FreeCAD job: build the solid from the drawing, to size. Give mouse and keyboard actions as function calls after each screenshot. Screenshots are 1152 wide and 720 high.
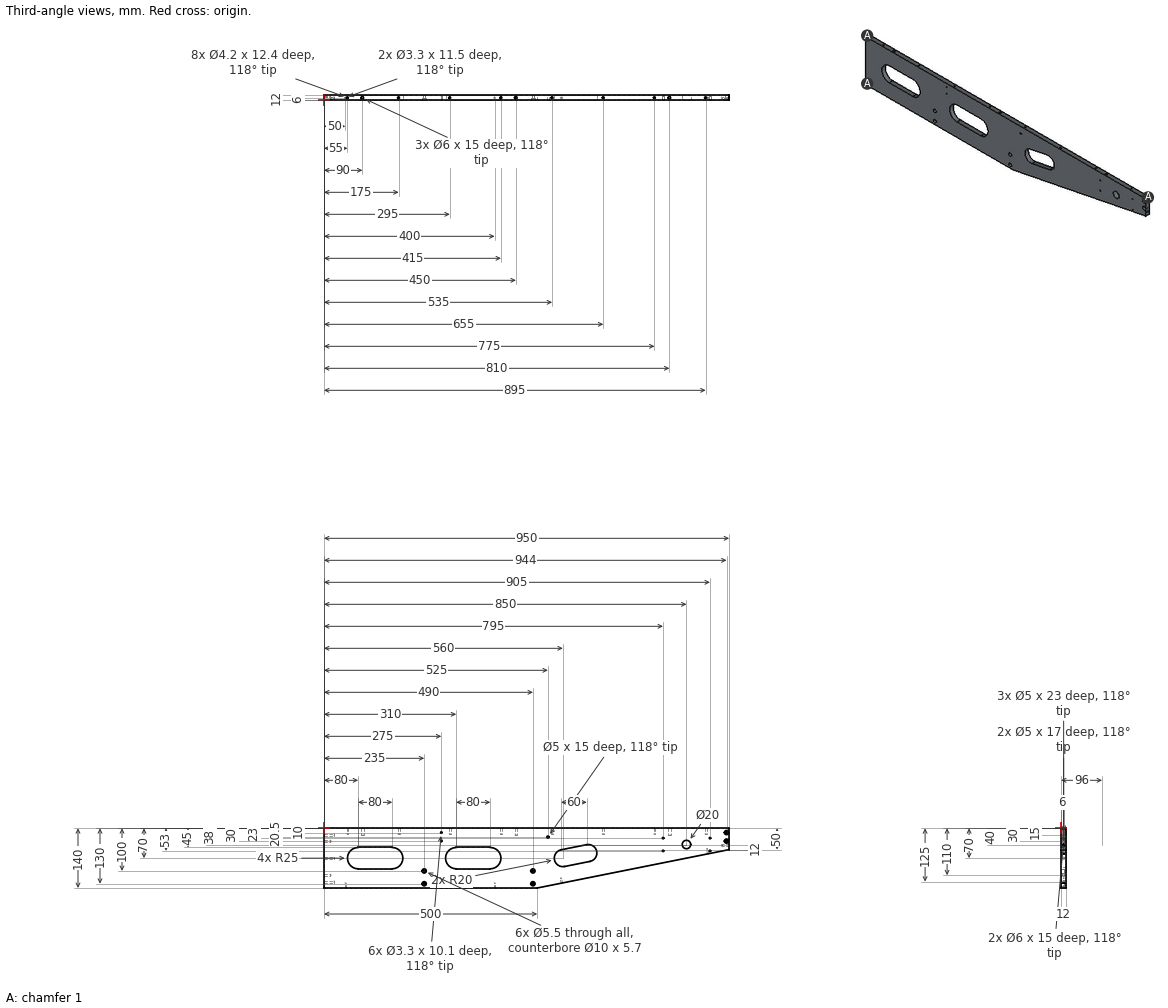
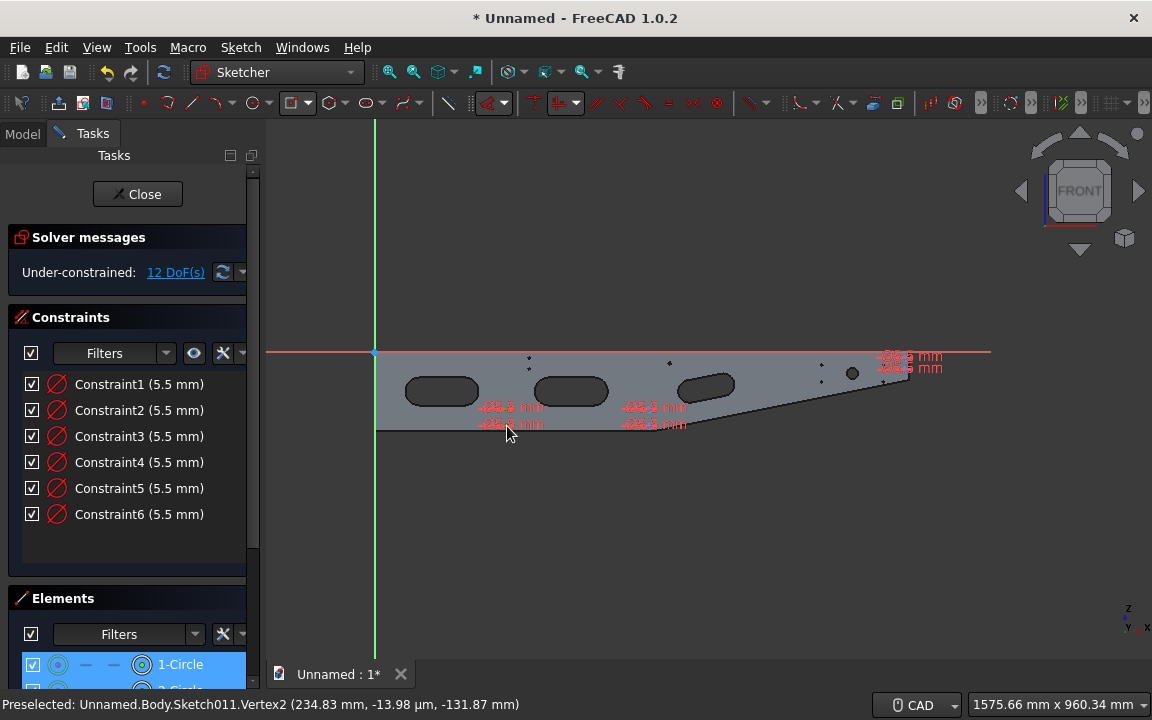
key(v)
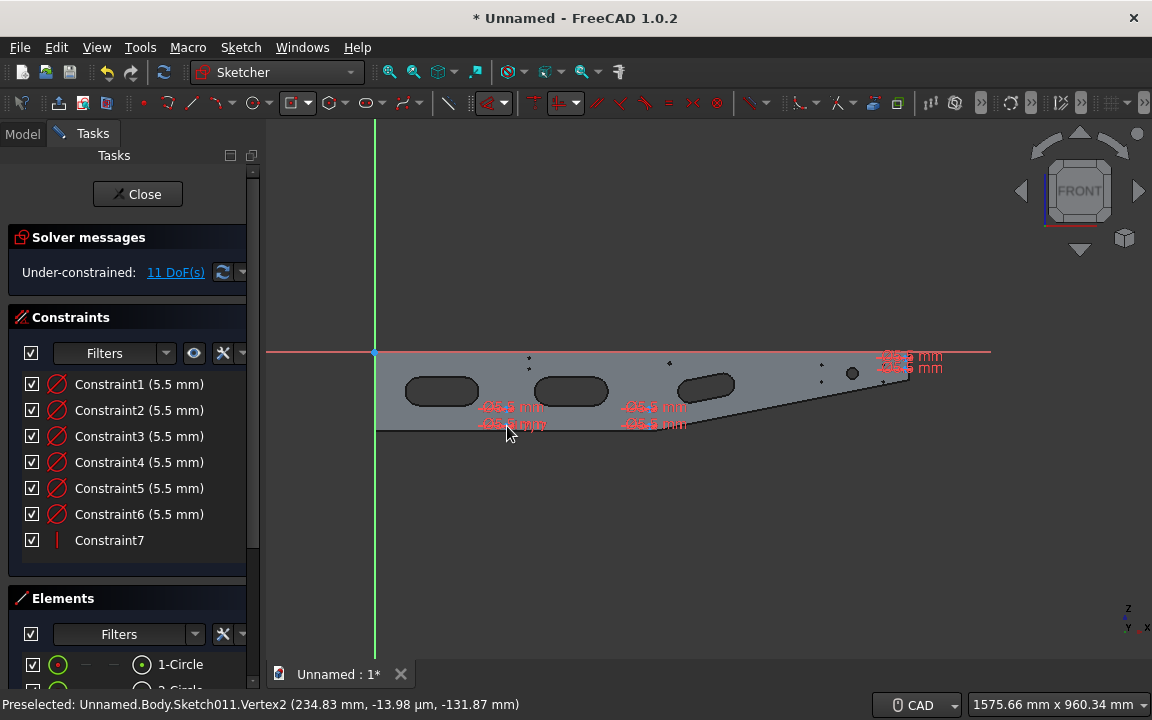
click(507, 409)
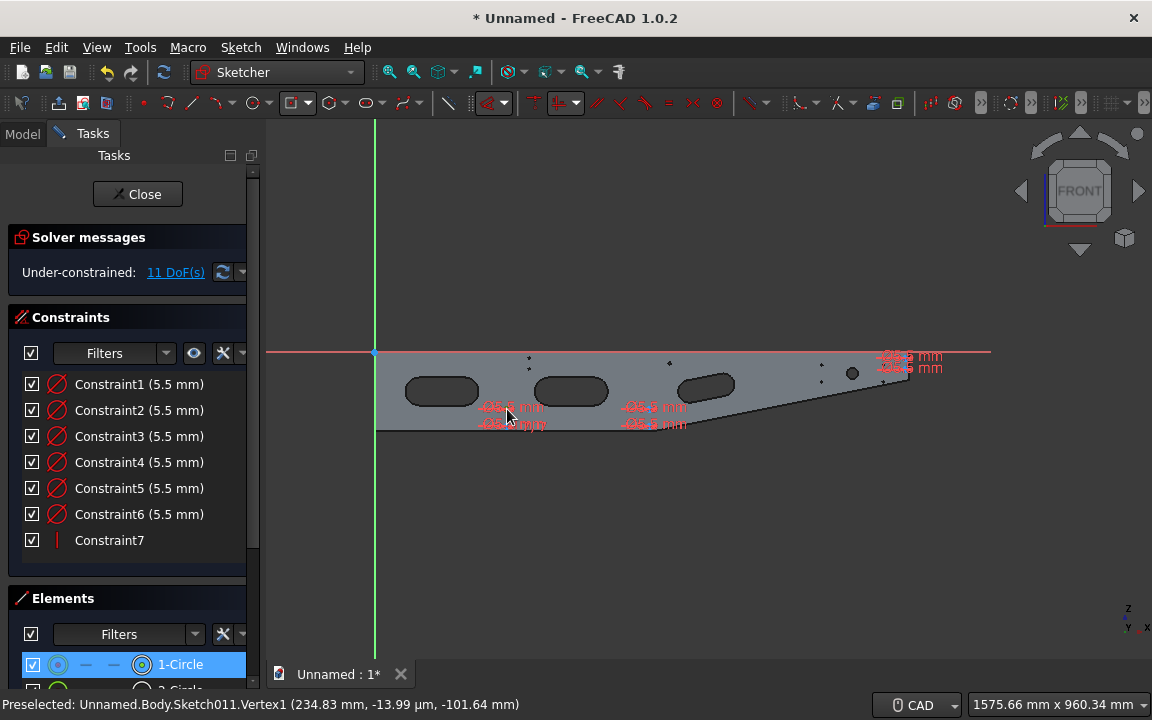
click(650, 409)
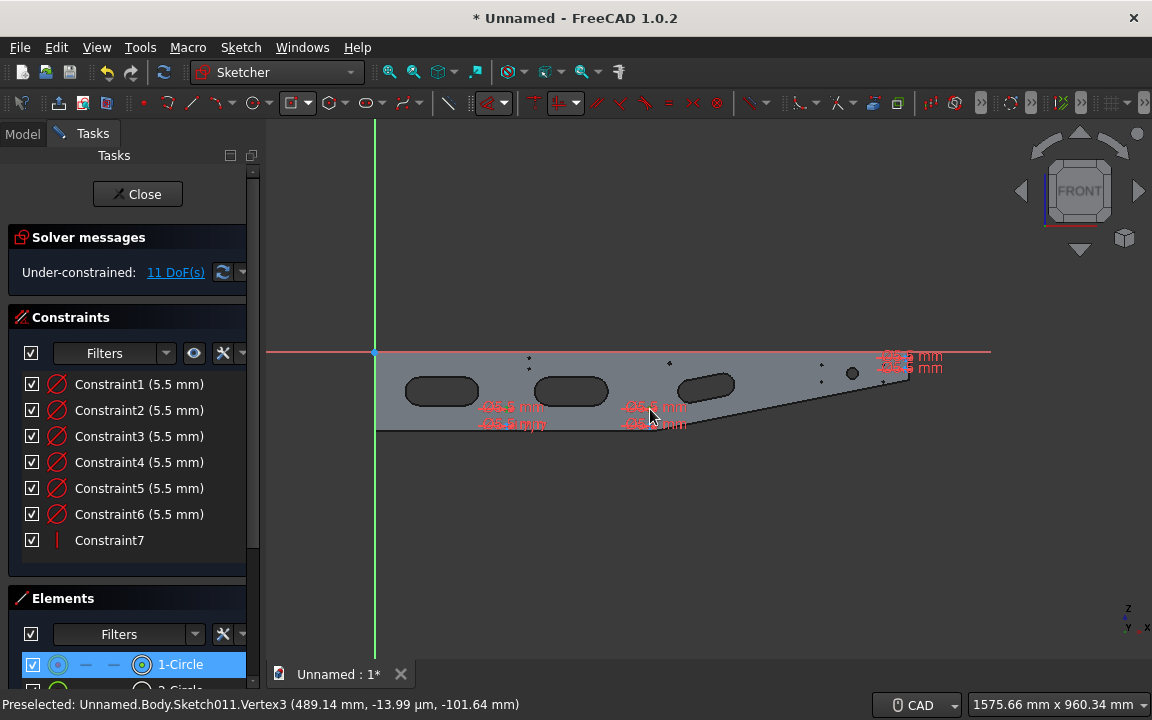
click(578, 104)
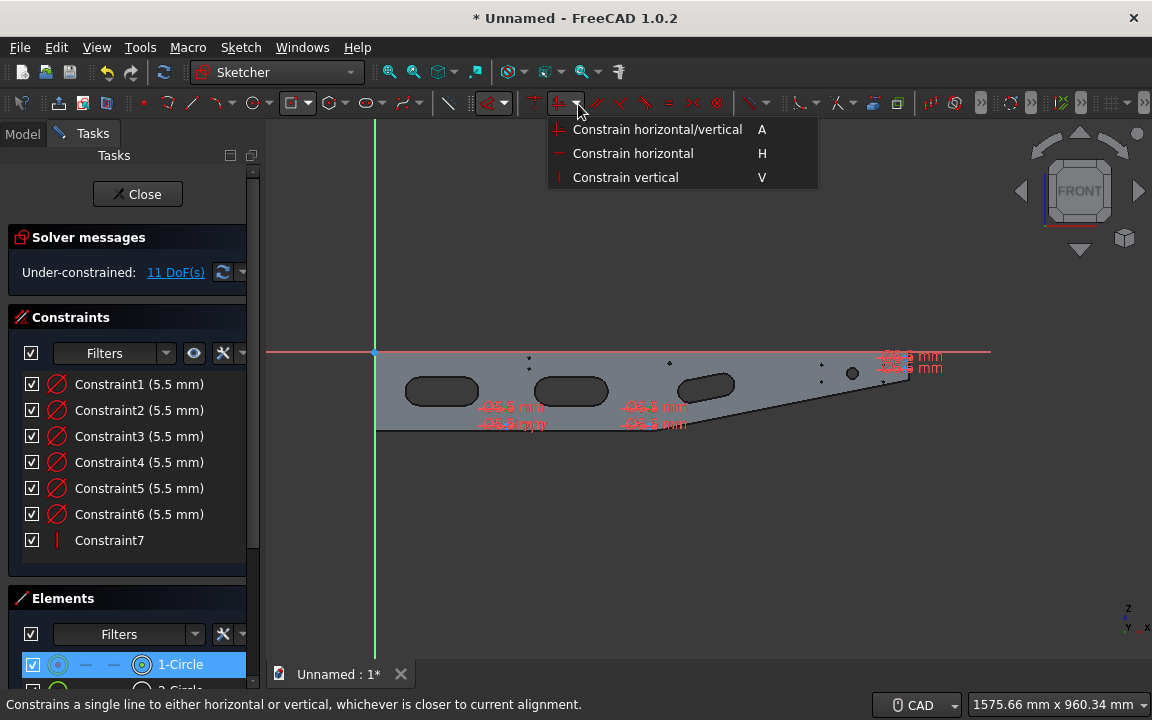
click(683, 153)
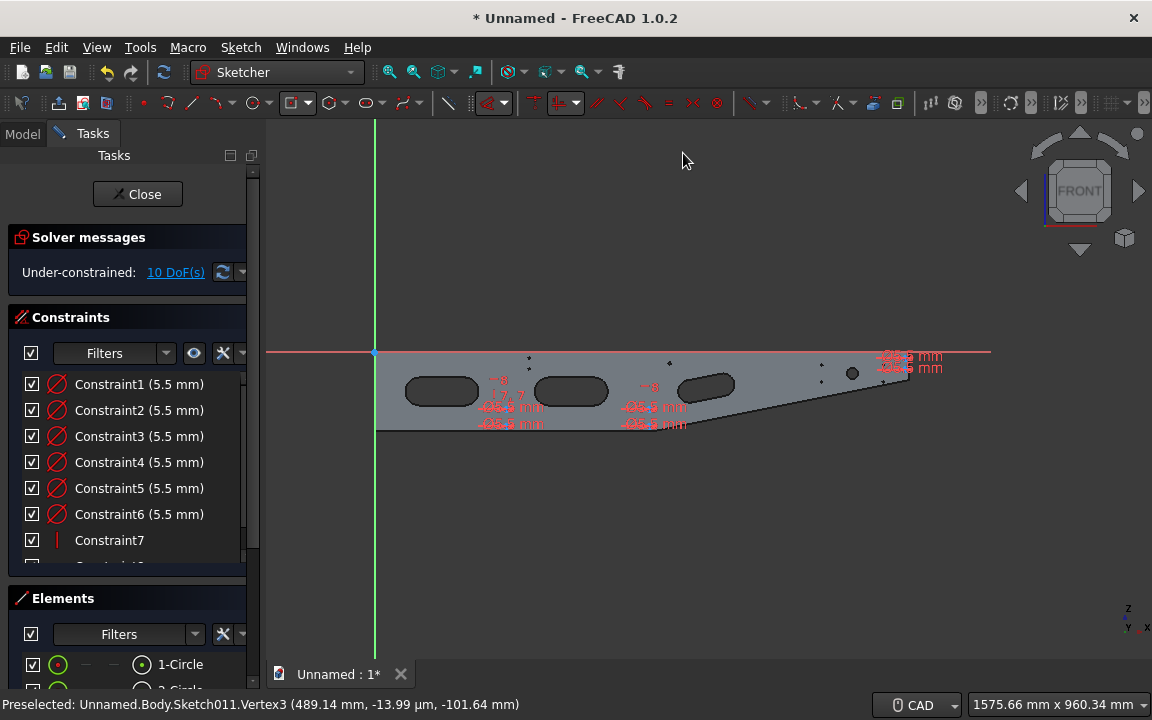
click(650, 409)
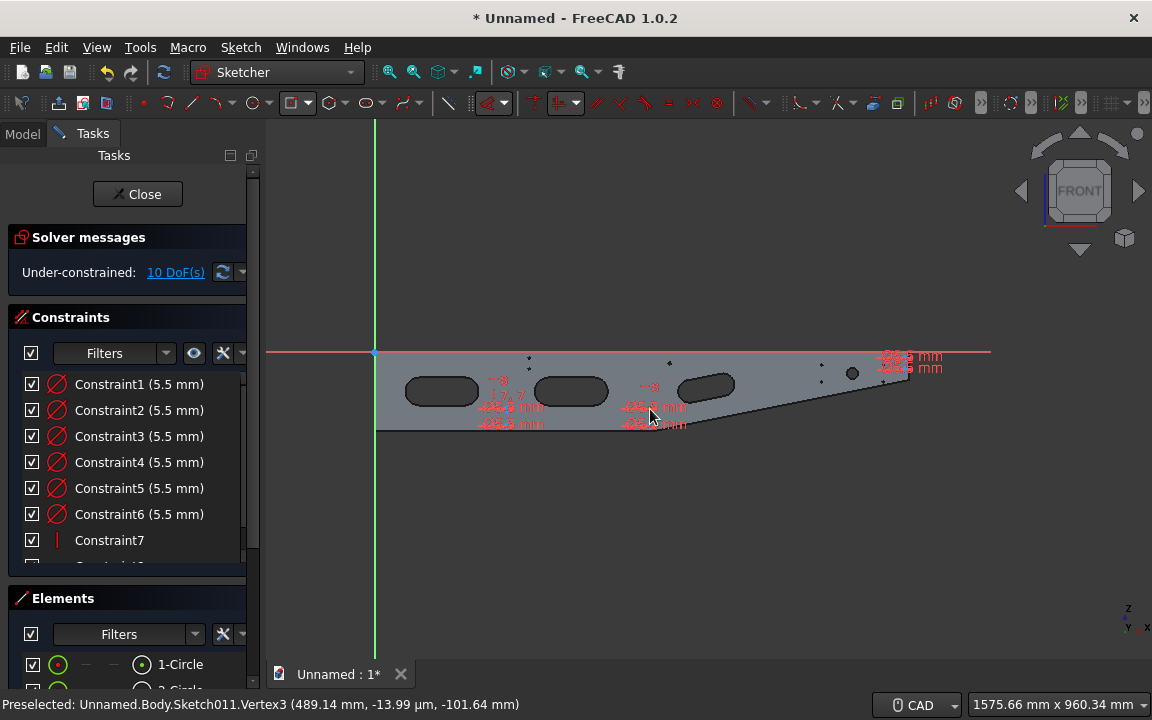
click(650, 426)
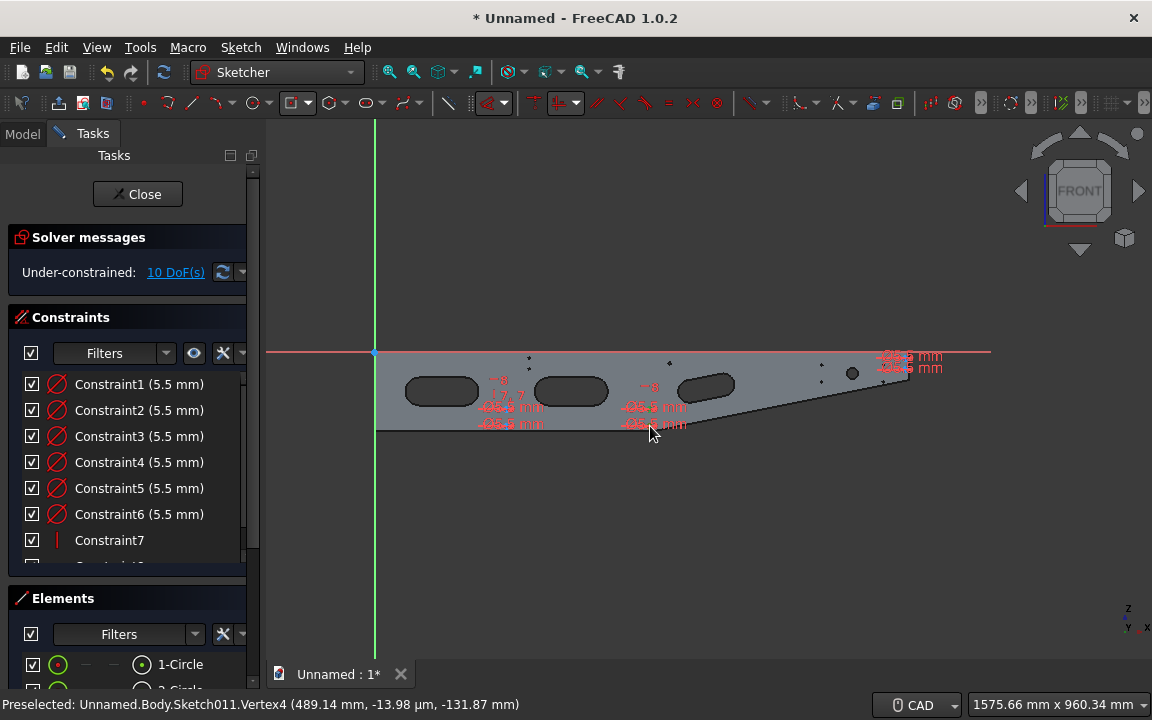
key(v)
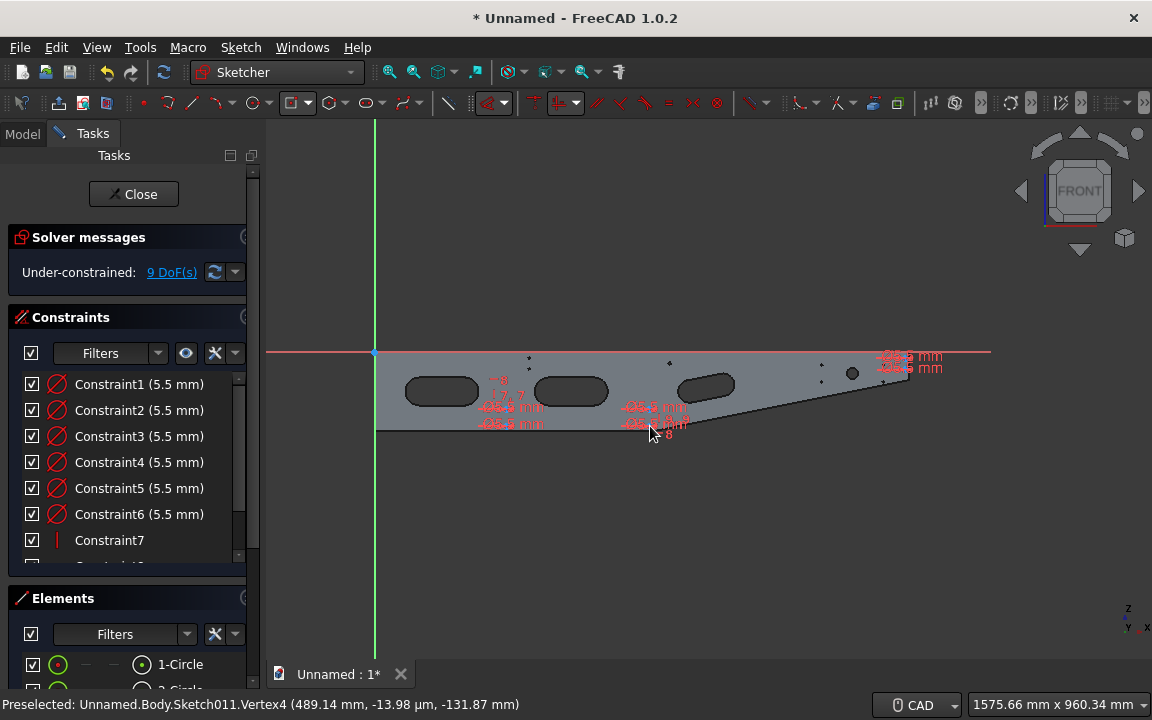
click(507, 426)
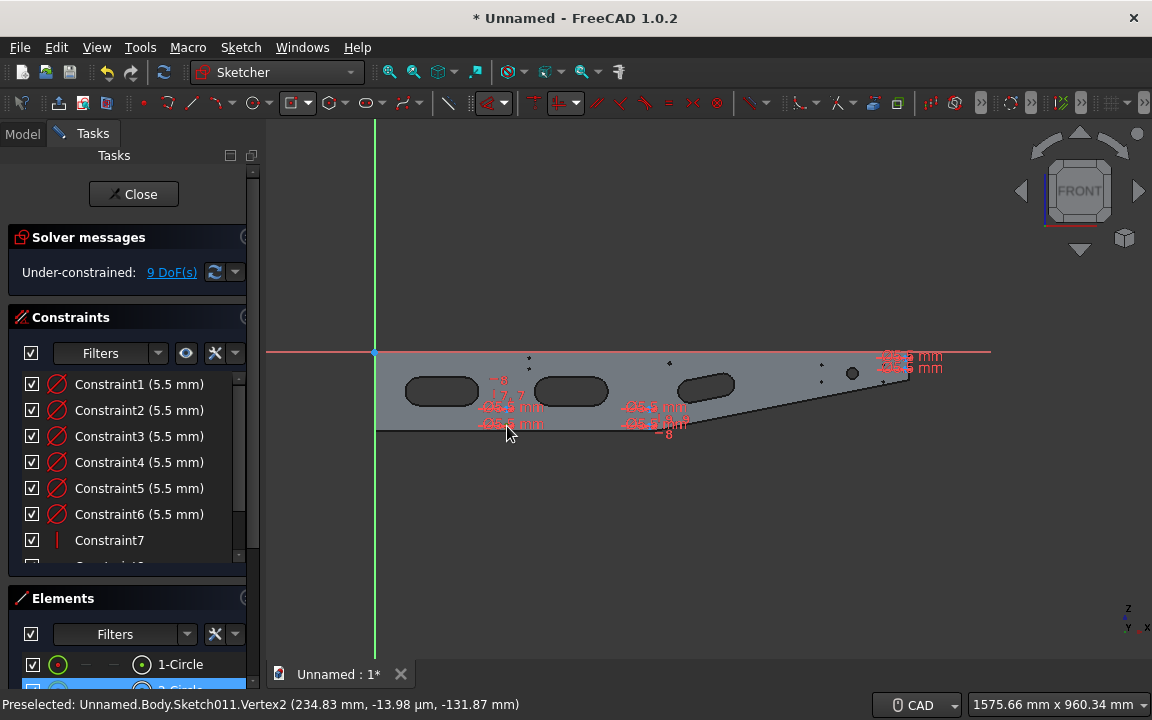
click(650, 426)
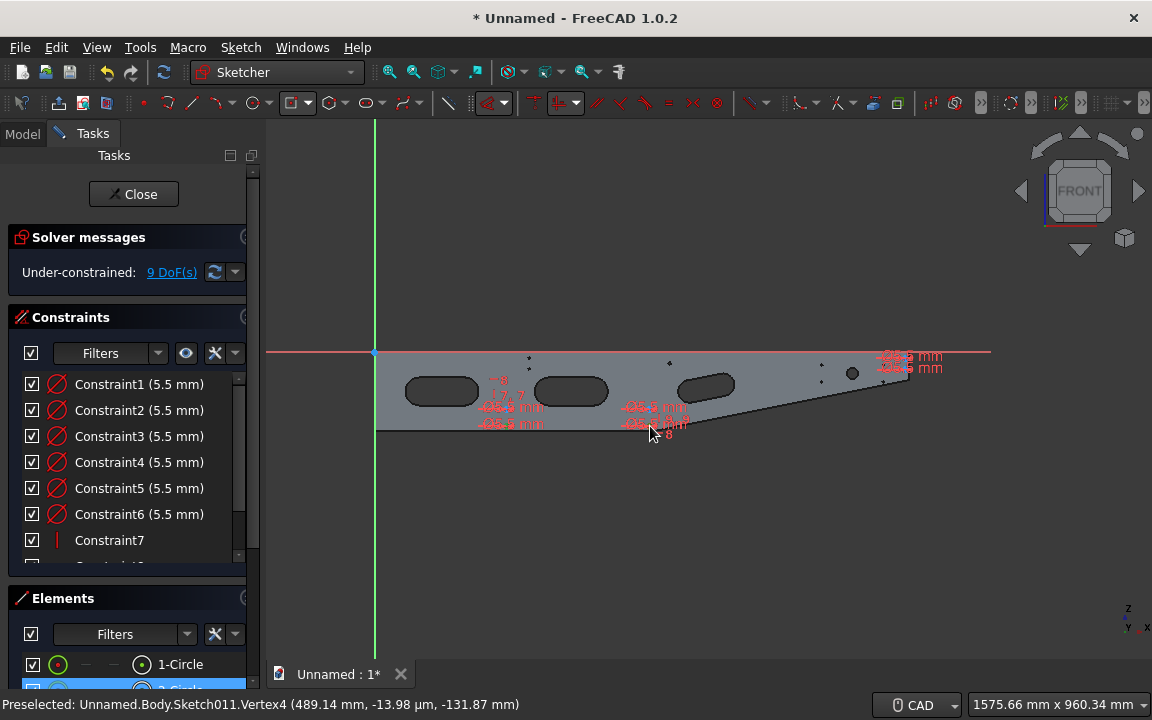
key(h)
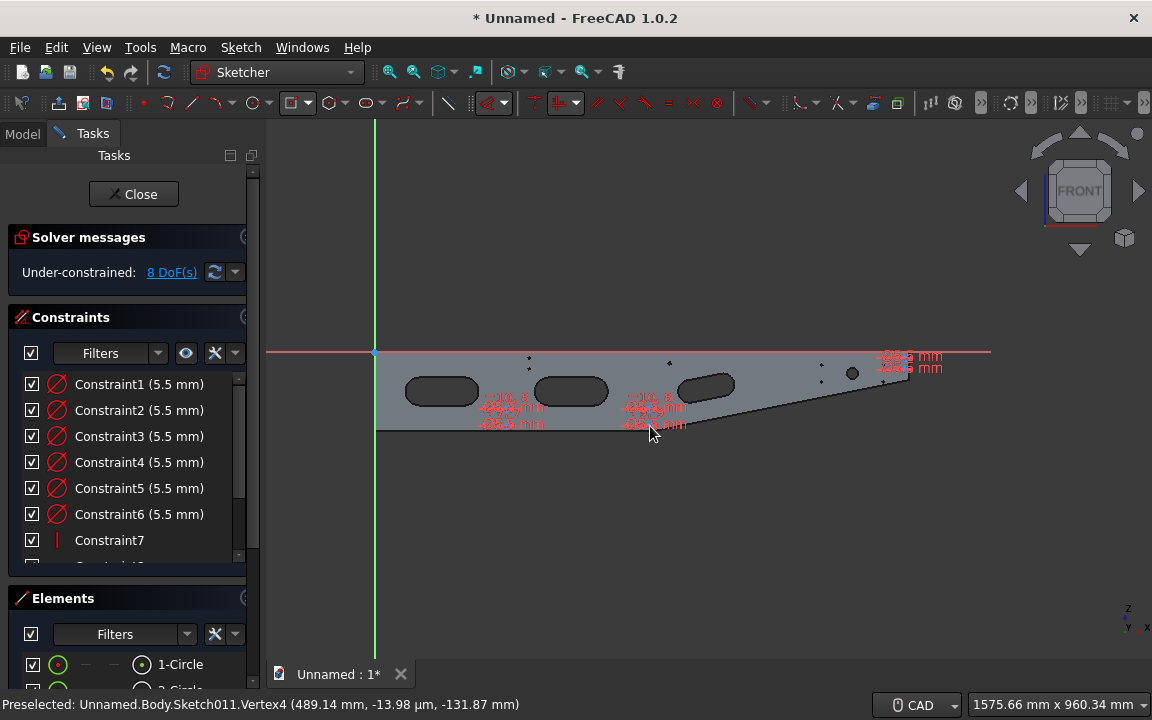
click(905, 358)